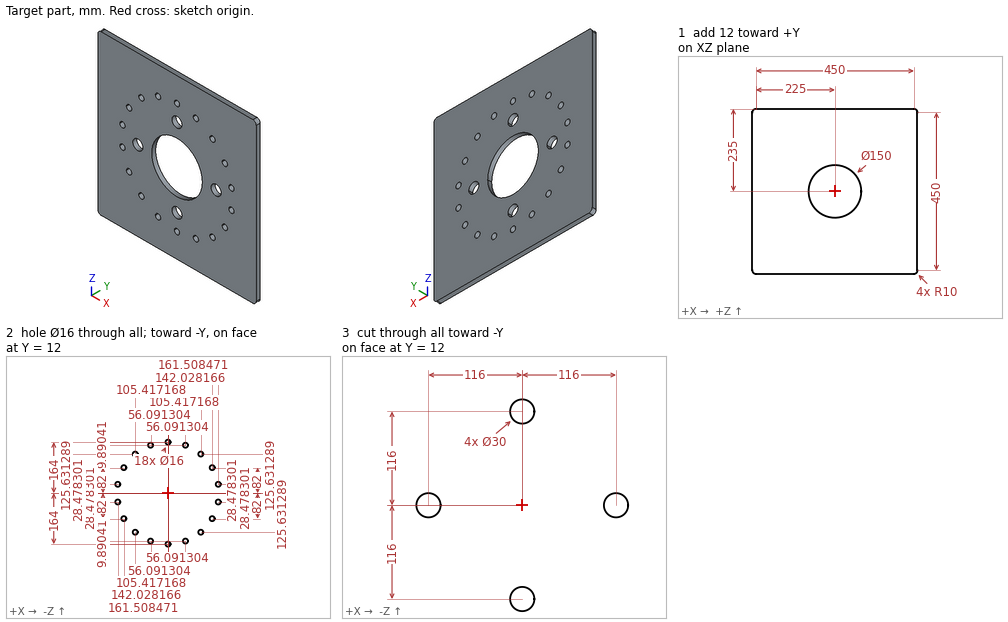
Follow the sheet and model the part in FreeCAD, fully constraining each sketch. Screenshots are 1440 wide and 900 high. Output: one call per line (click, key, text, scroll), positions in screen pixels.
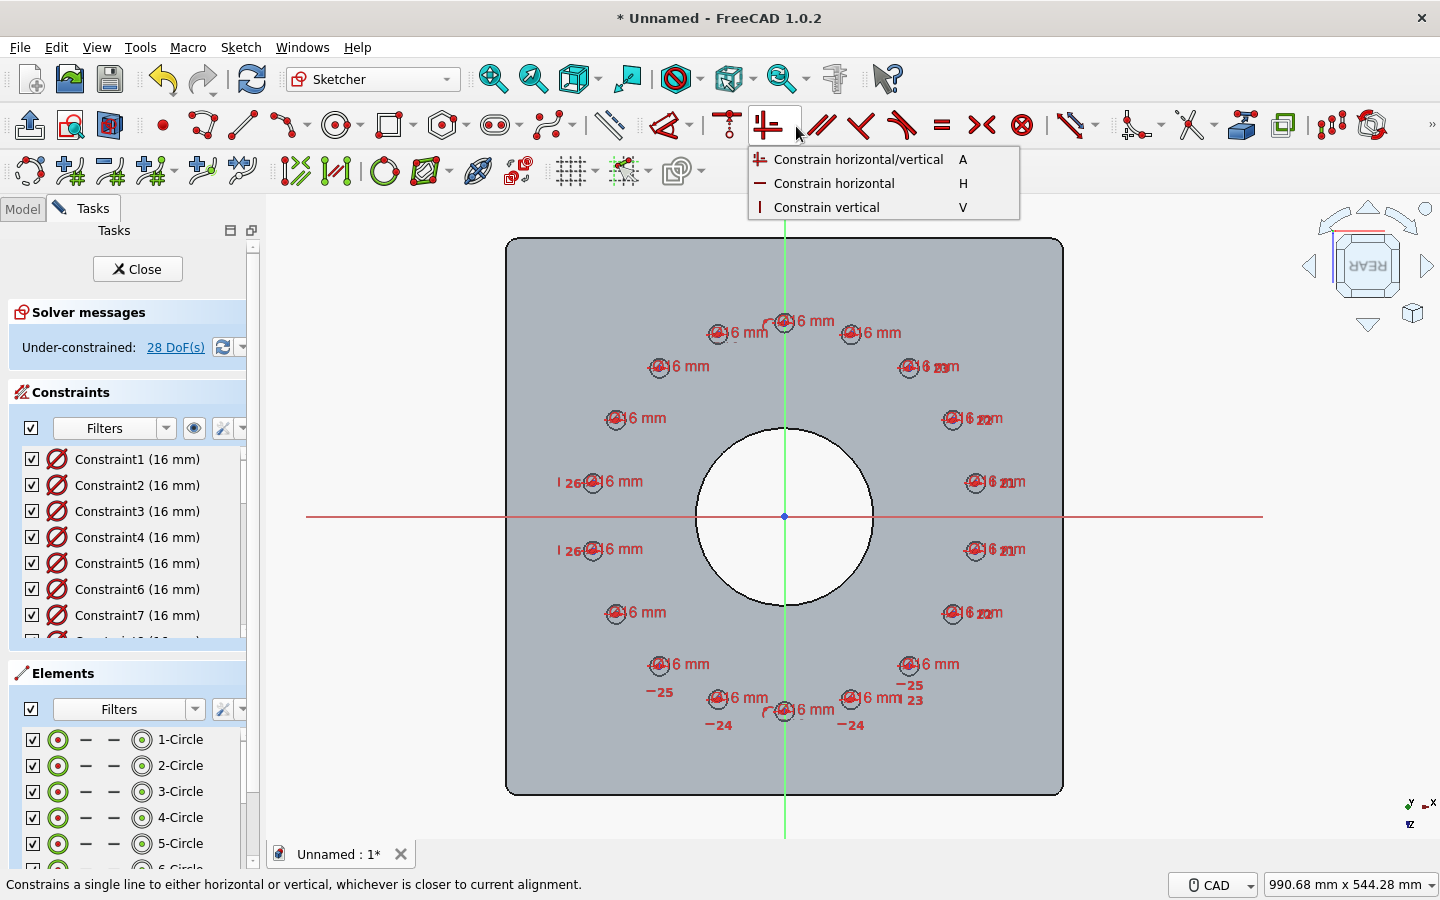
click(884, 207)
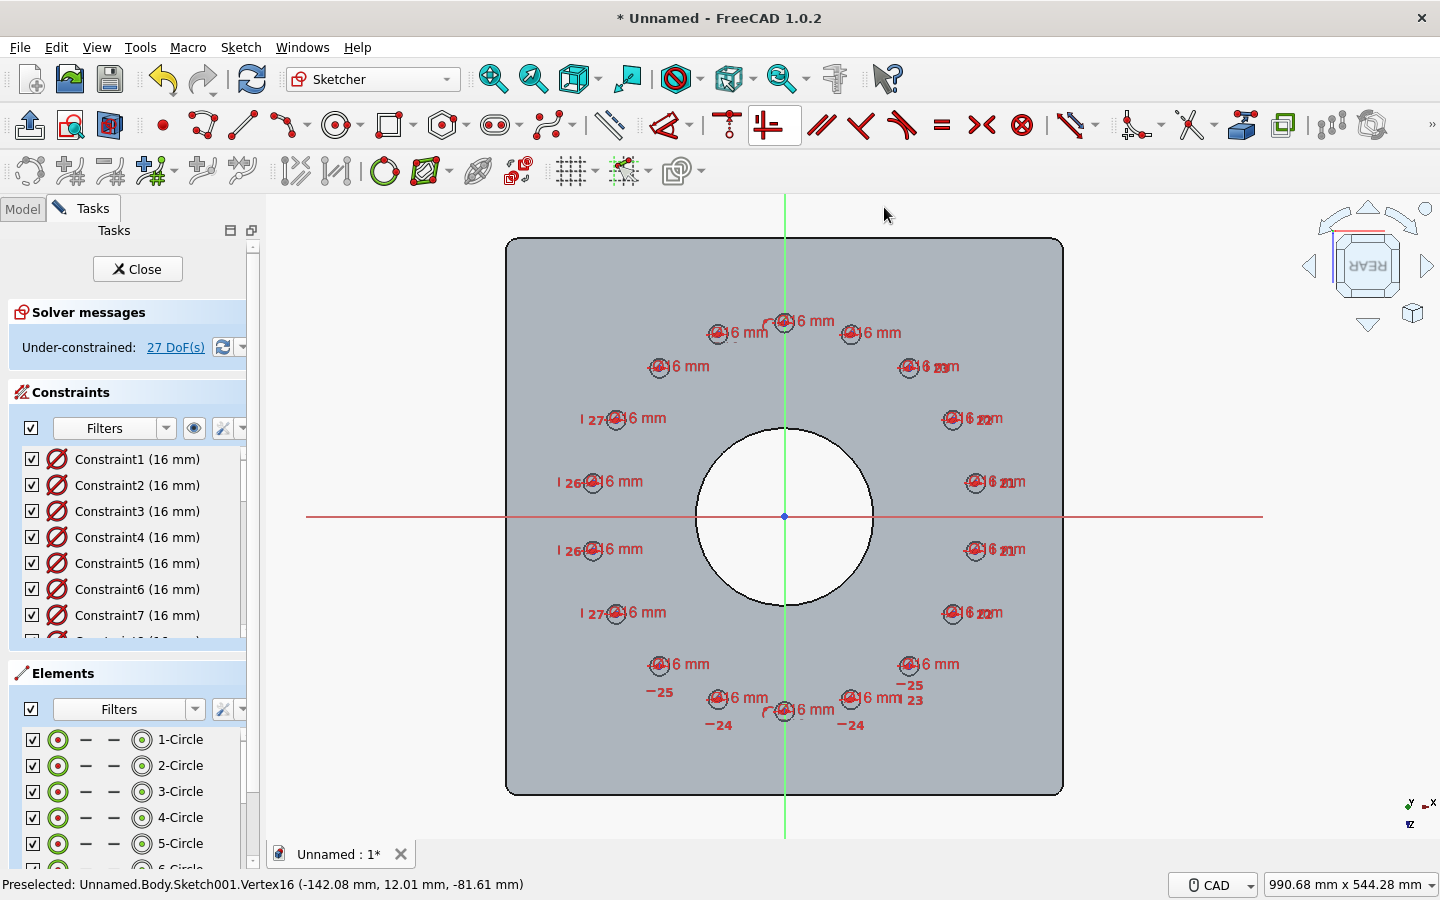
click(851, 335)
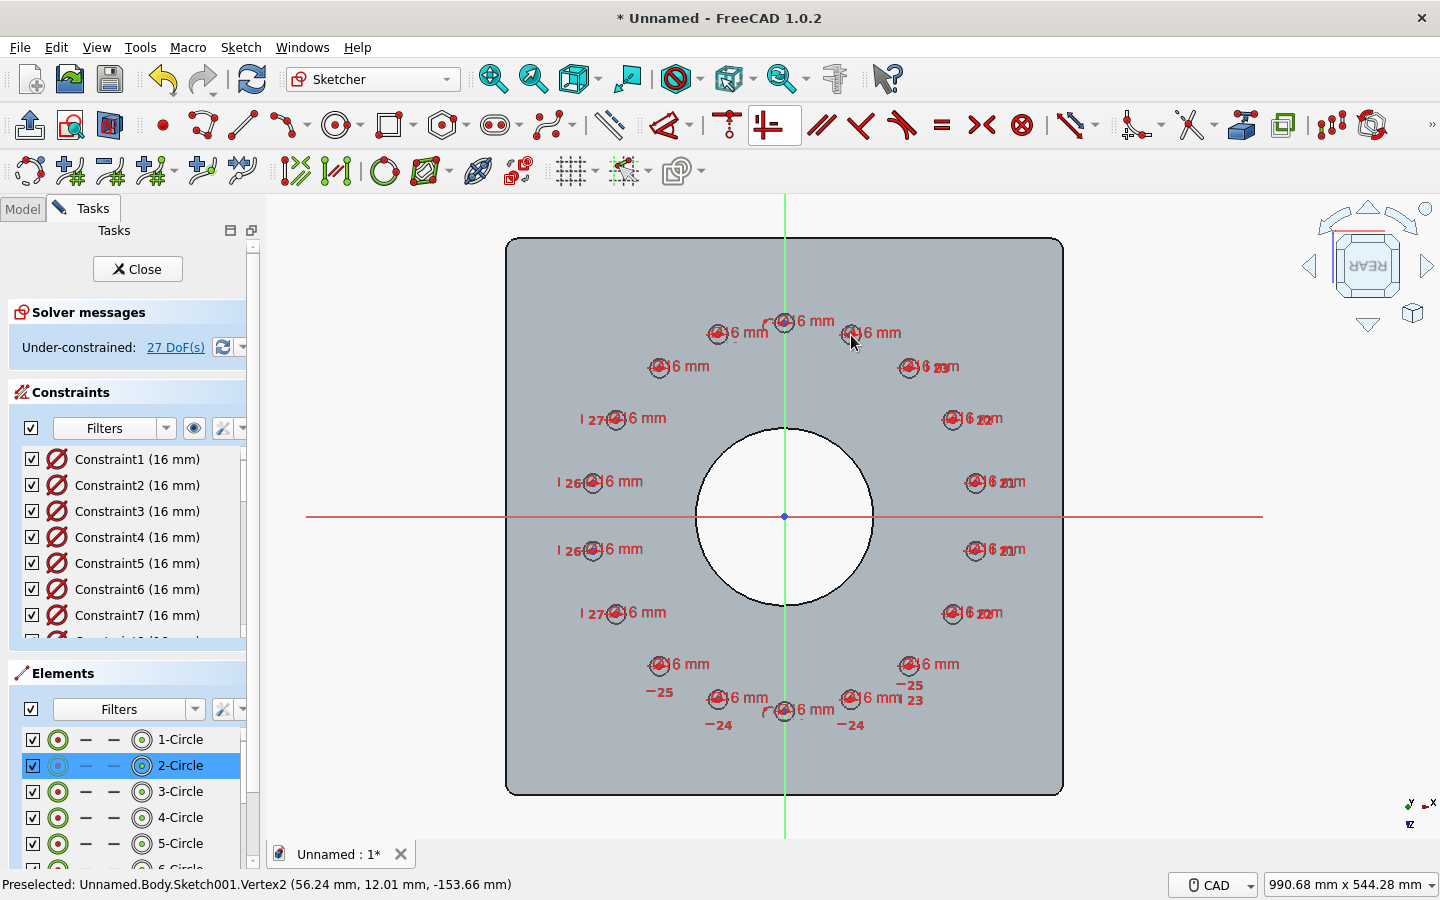
click(718, 335)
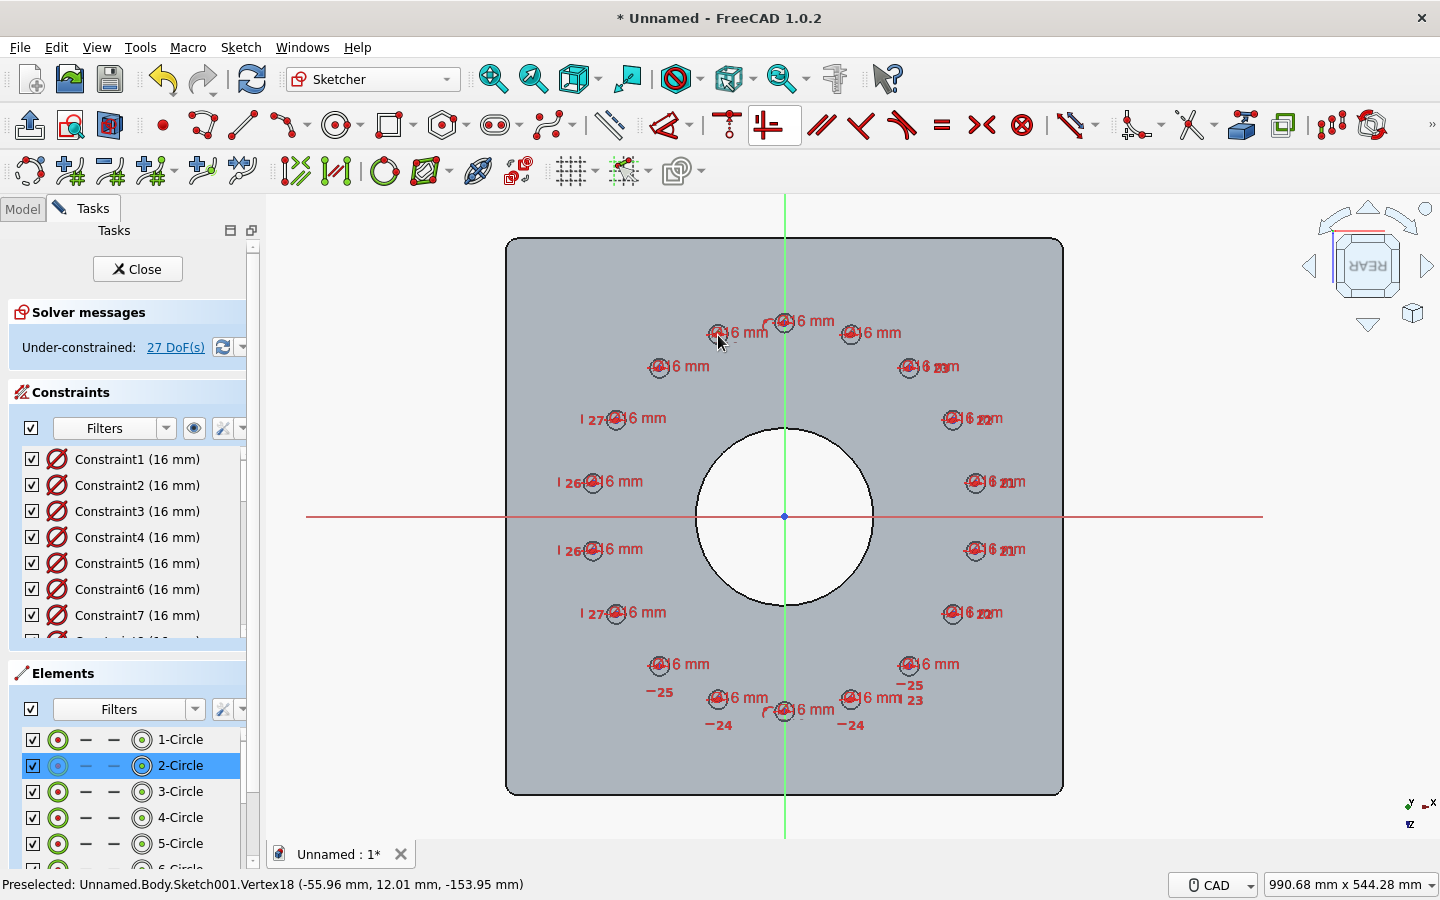
click(796, 126)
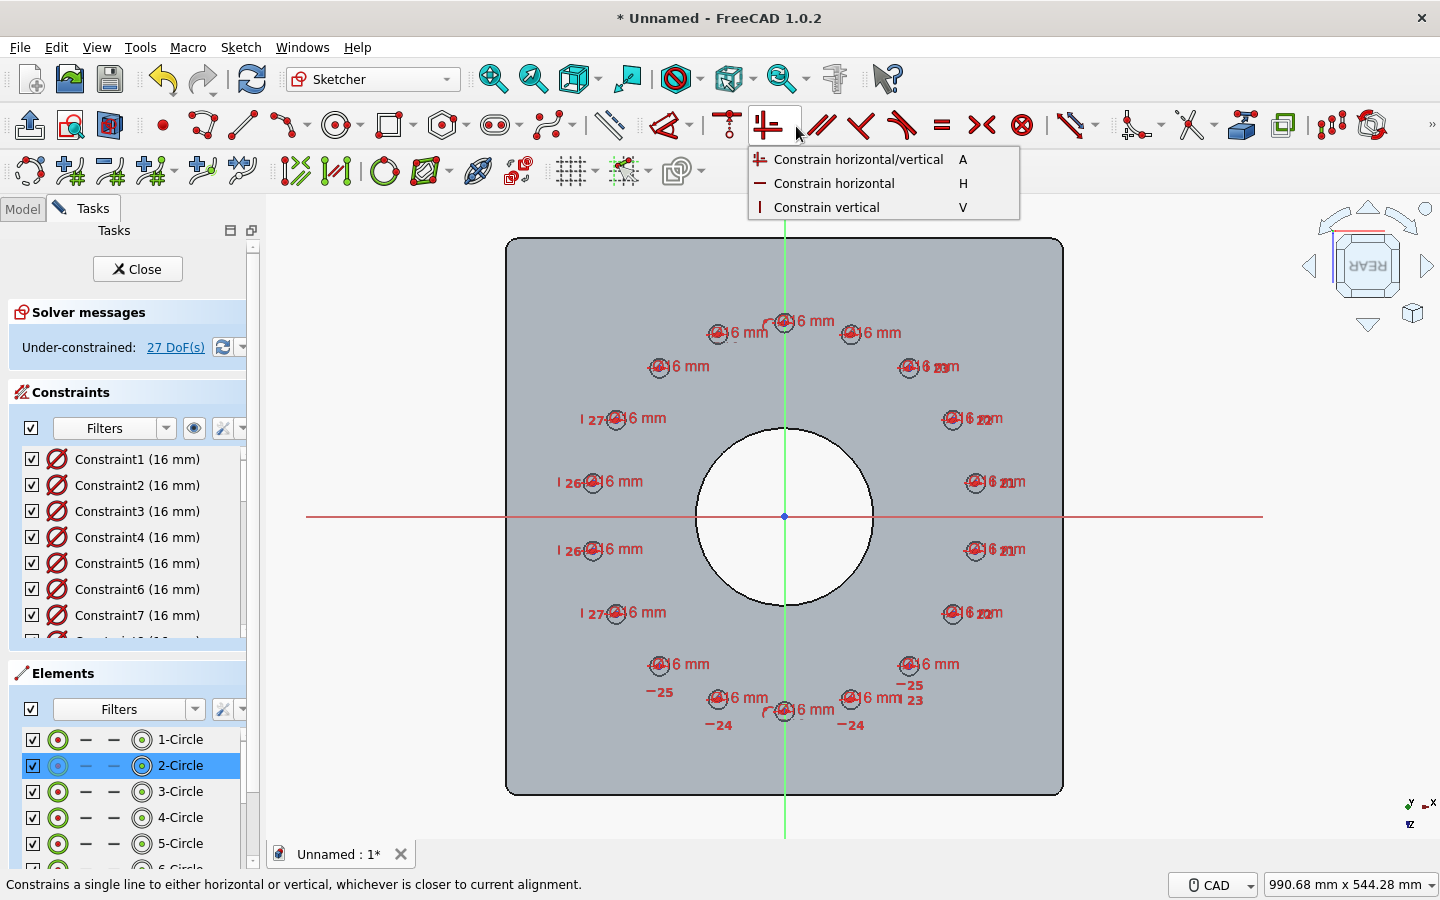
click(884, 183)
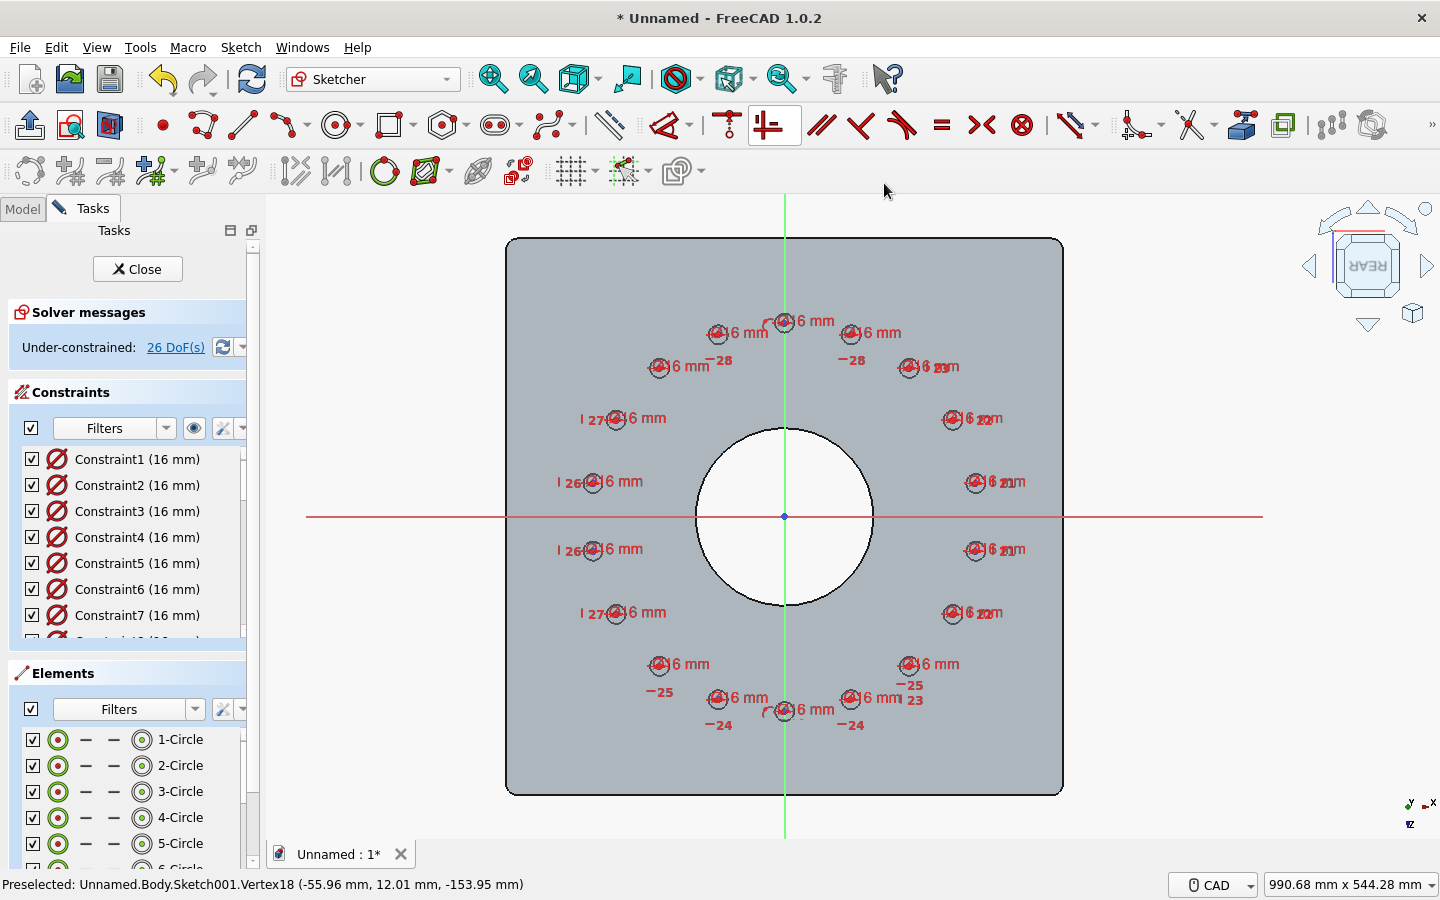
click(664, 126)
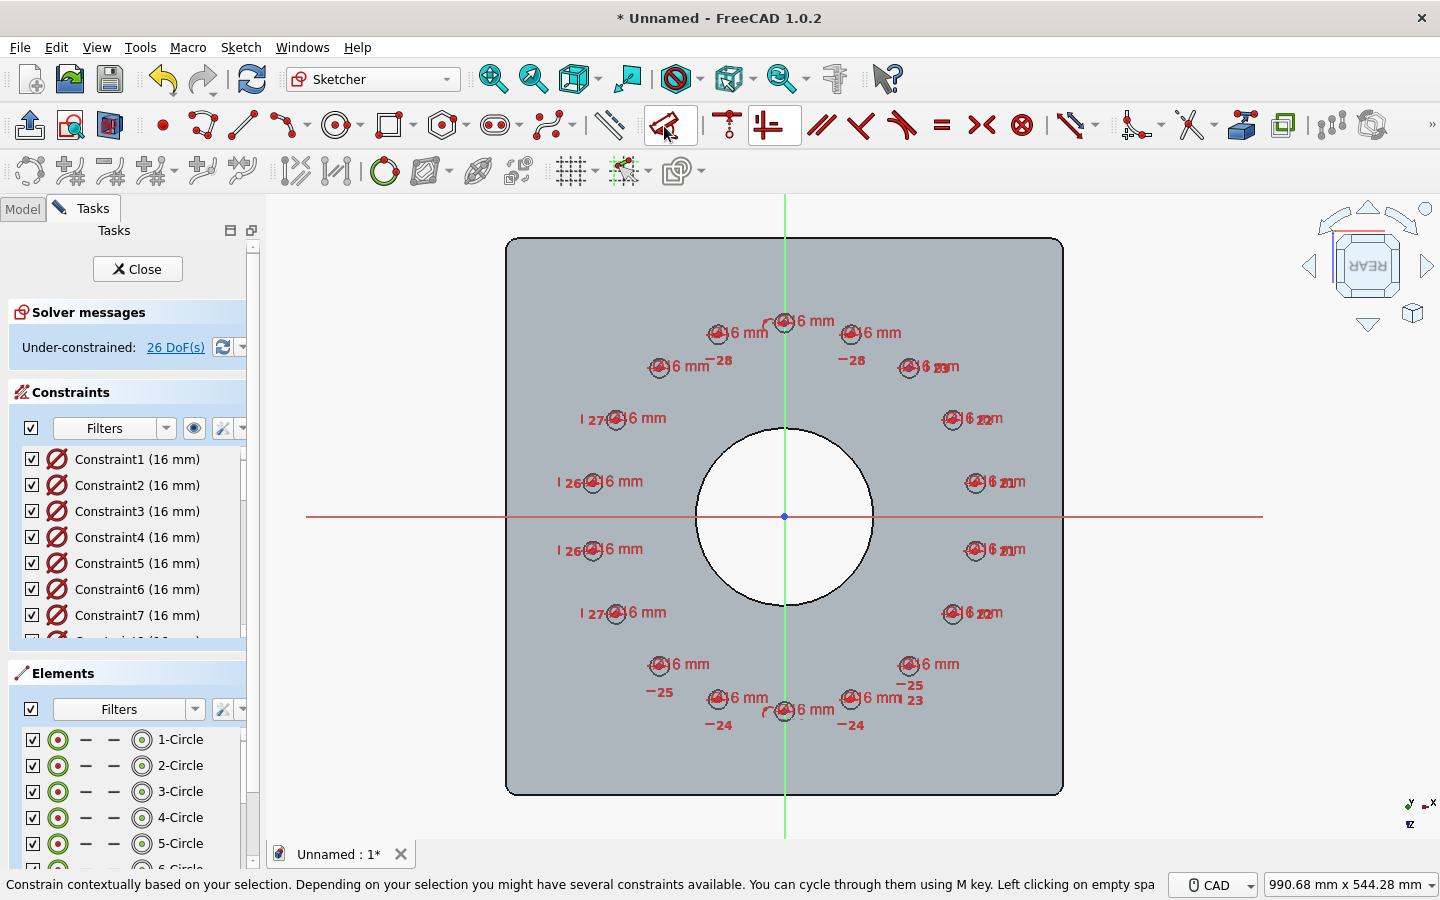
click(953, 420)
click(987, 446)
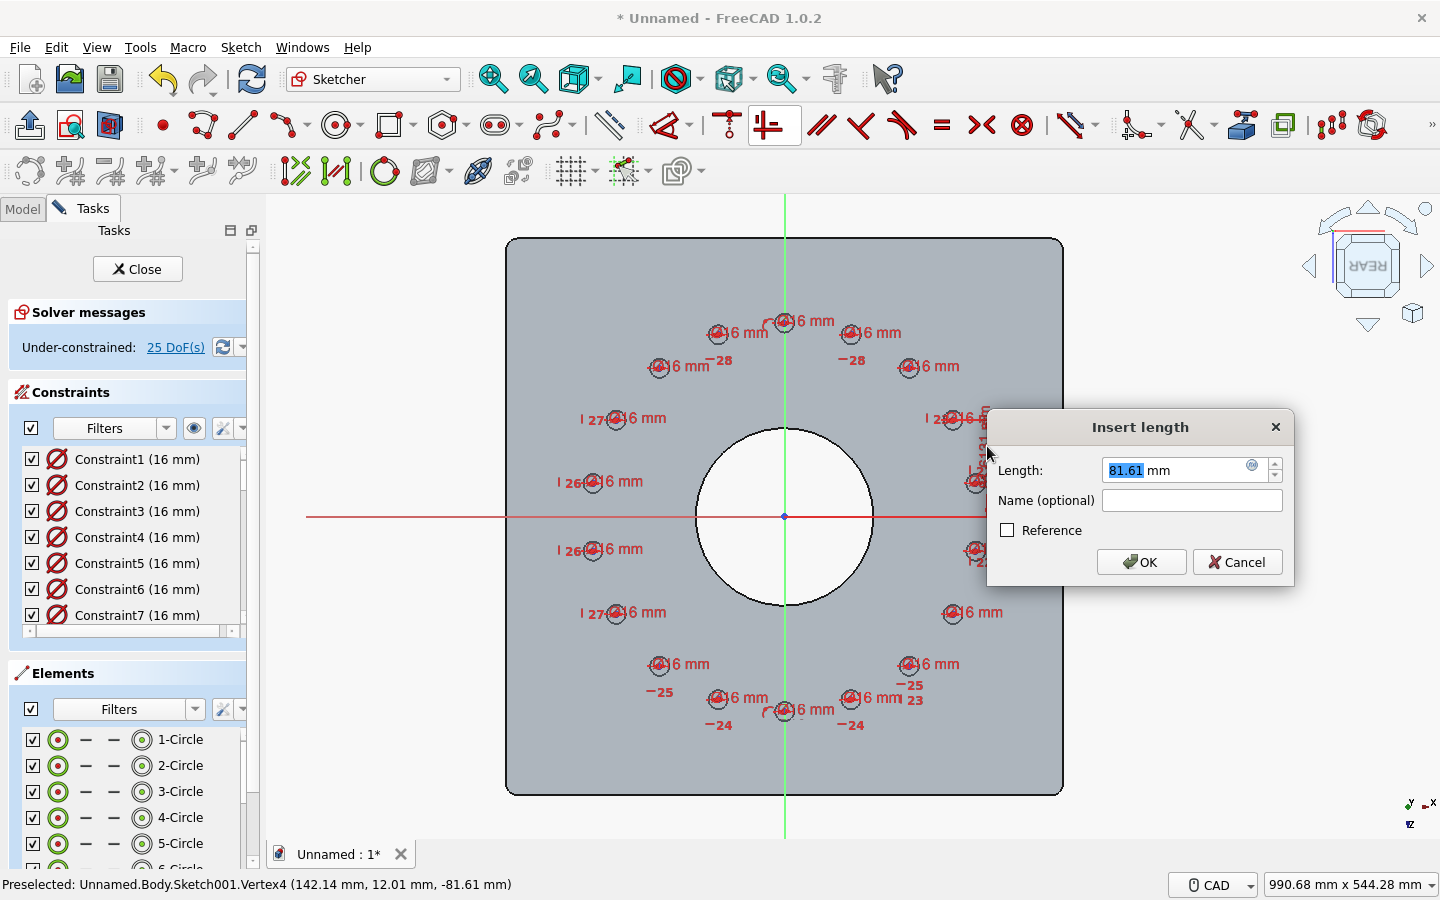
text(82)
key(Return)